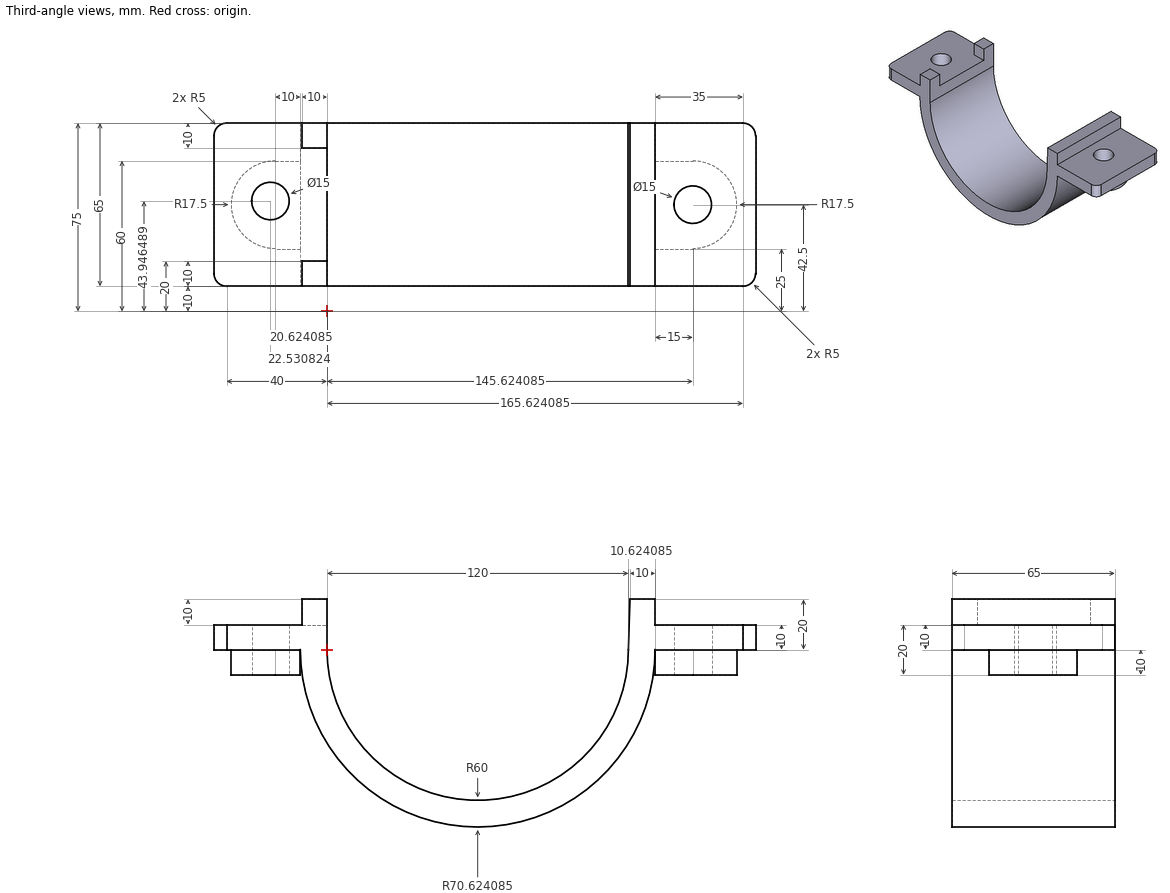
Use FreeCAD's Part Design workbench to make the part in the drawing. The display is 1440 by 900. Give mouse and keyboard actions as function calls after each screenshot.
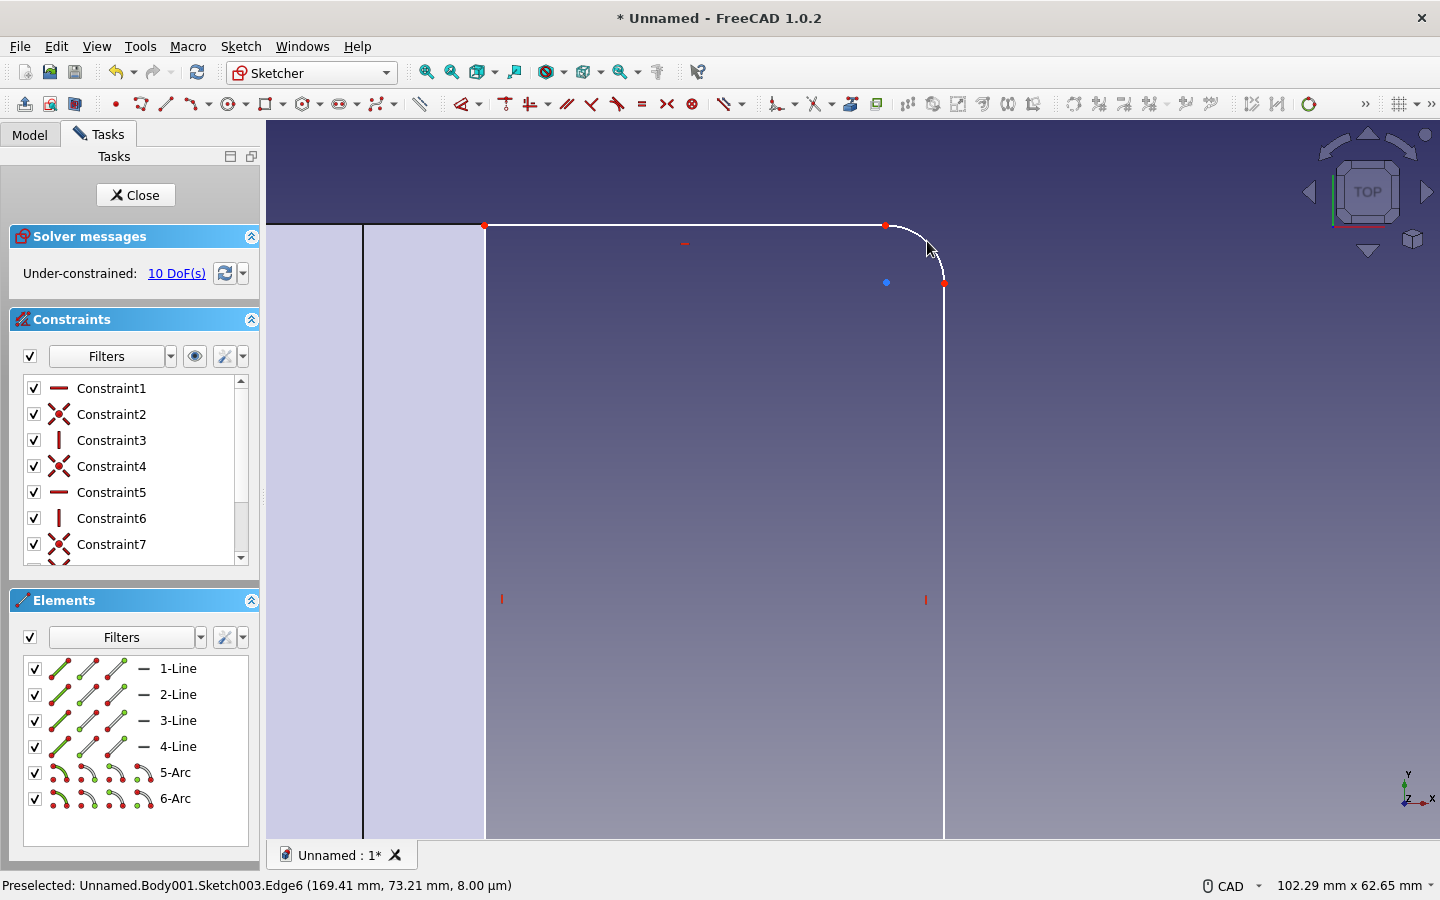
click(766, 225)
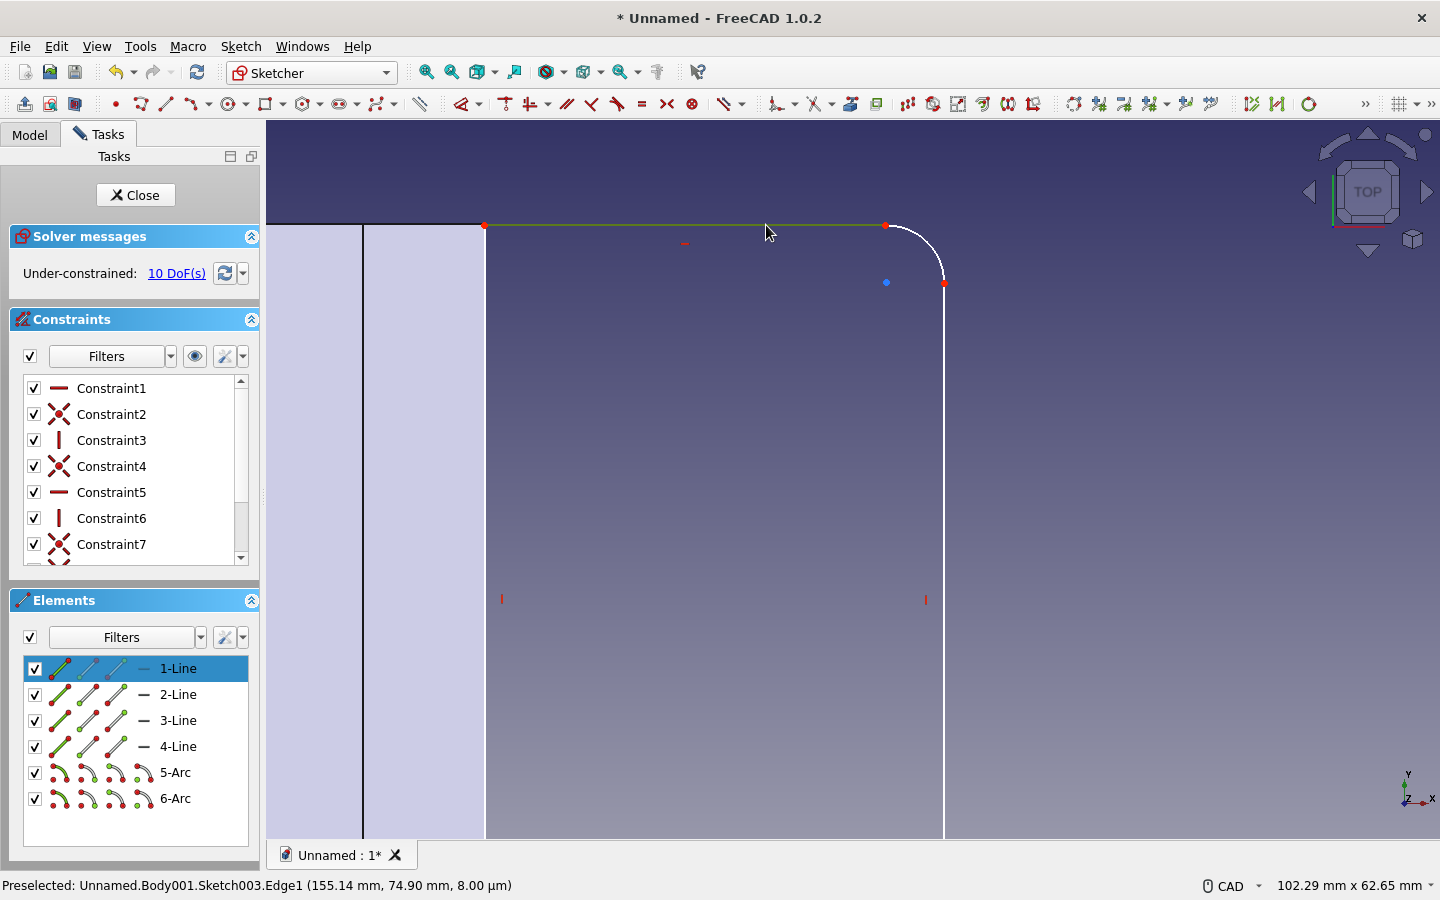
click(938, 257)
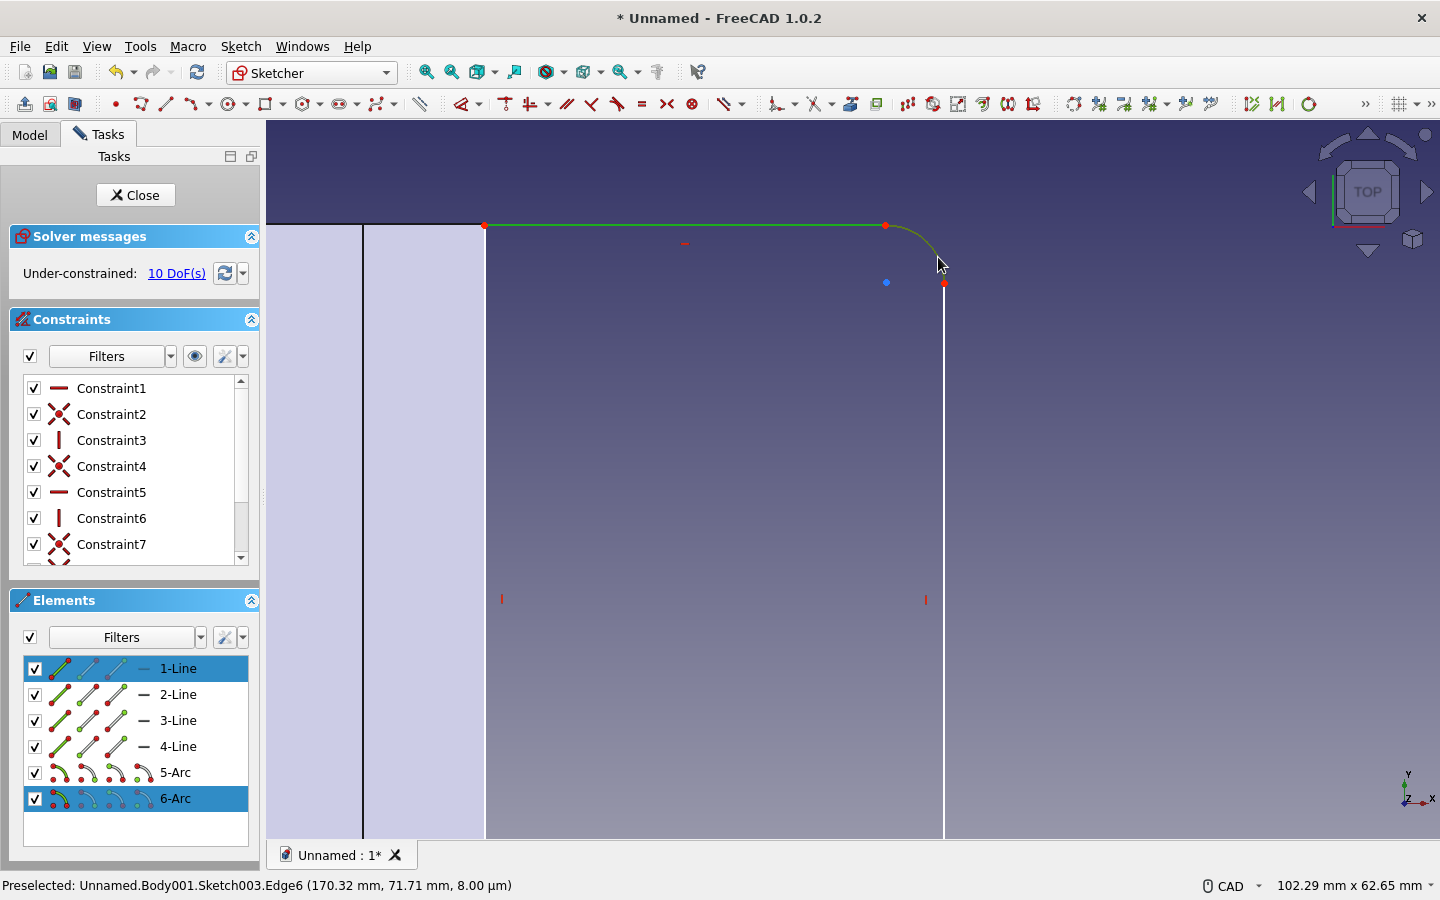
key(t)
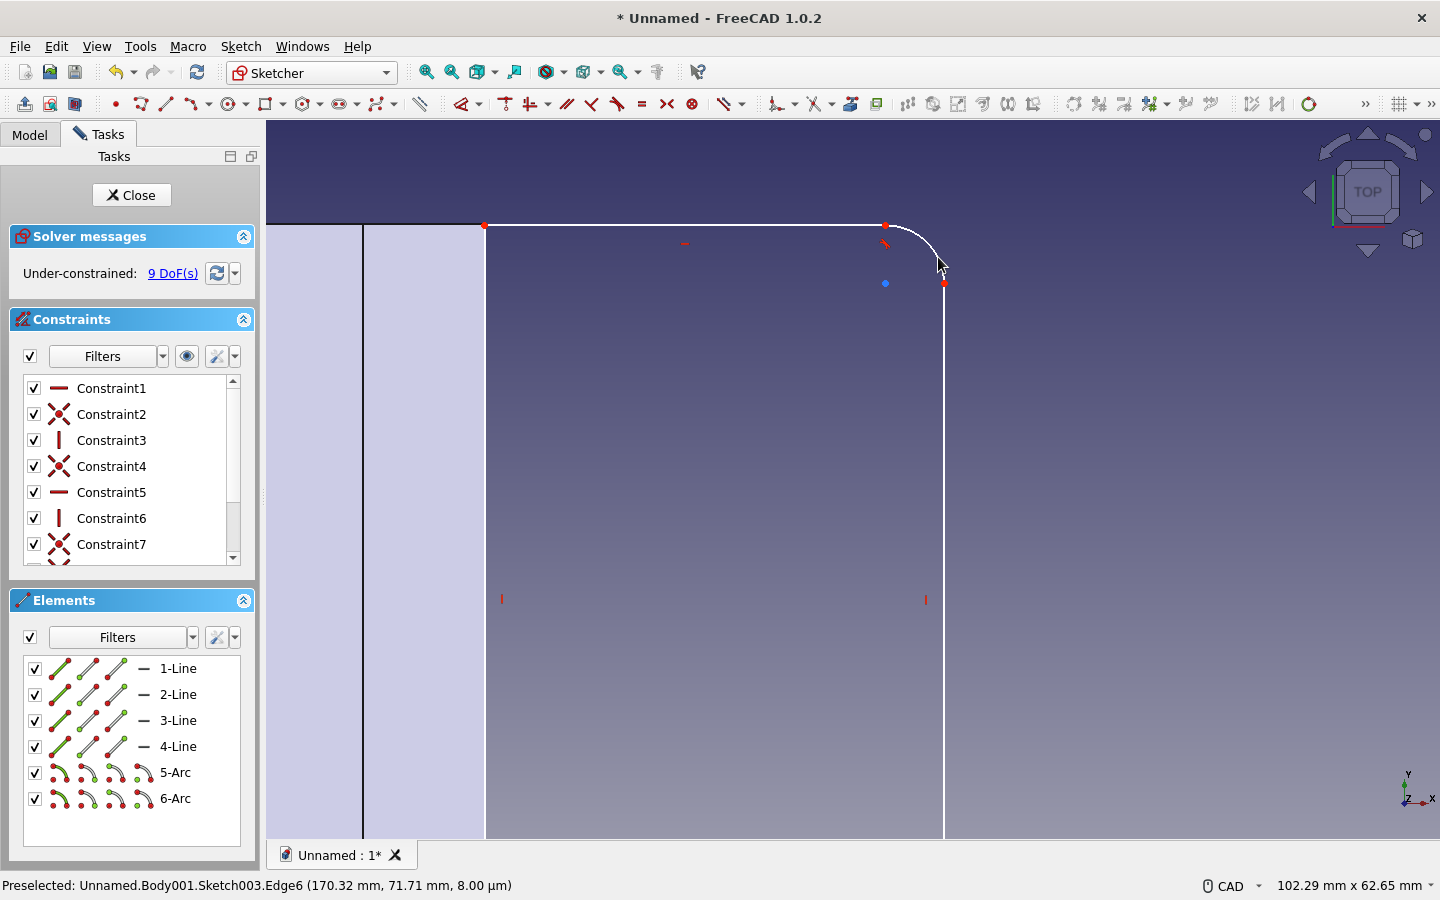
scroll(927, 240, down, 2)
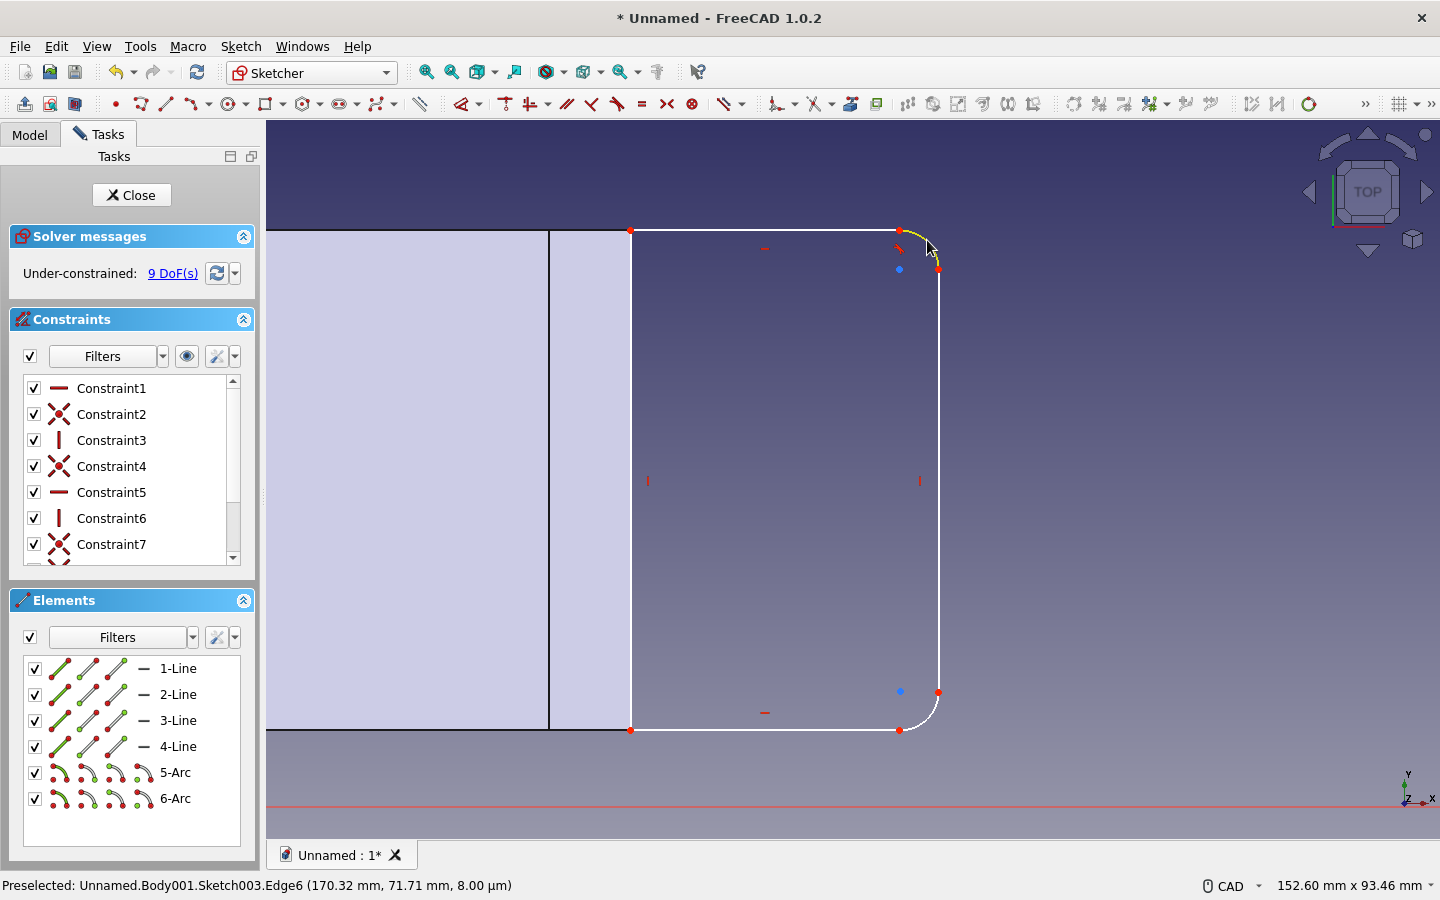
click(711, 730)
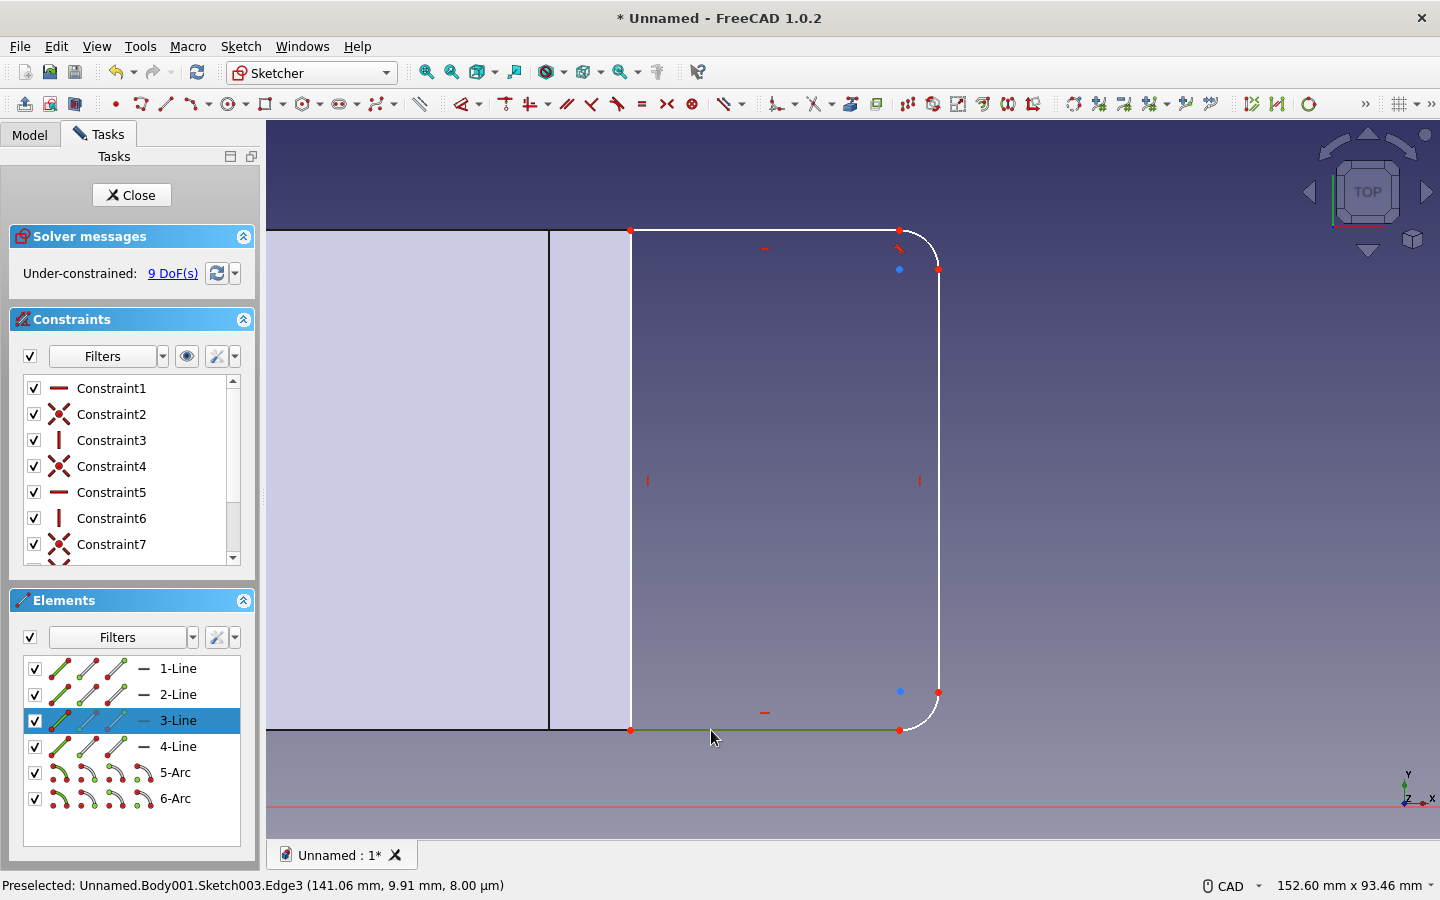
click(917, 726)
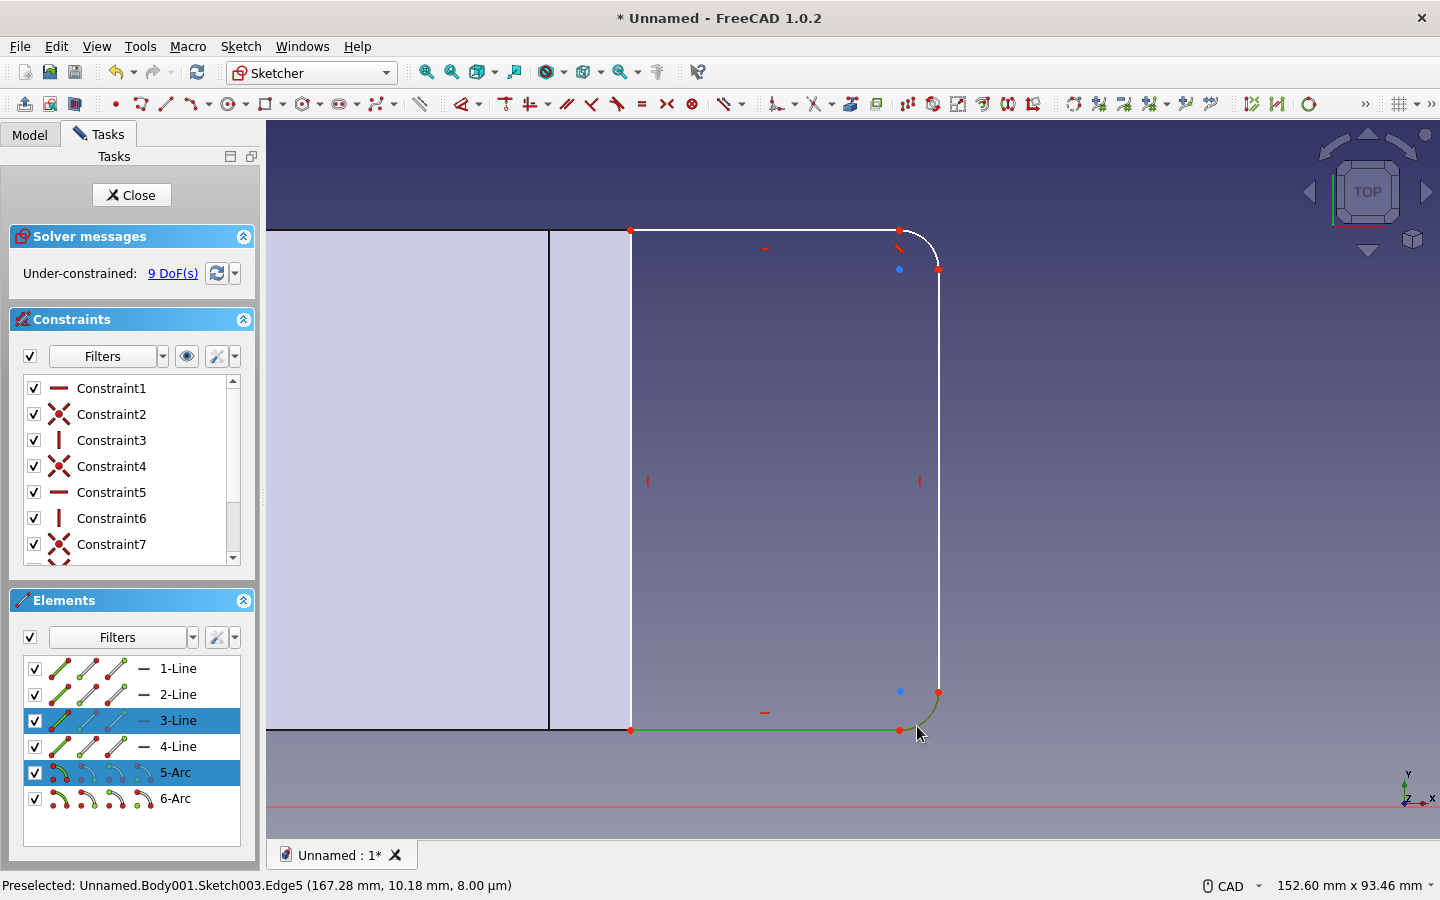
key(t)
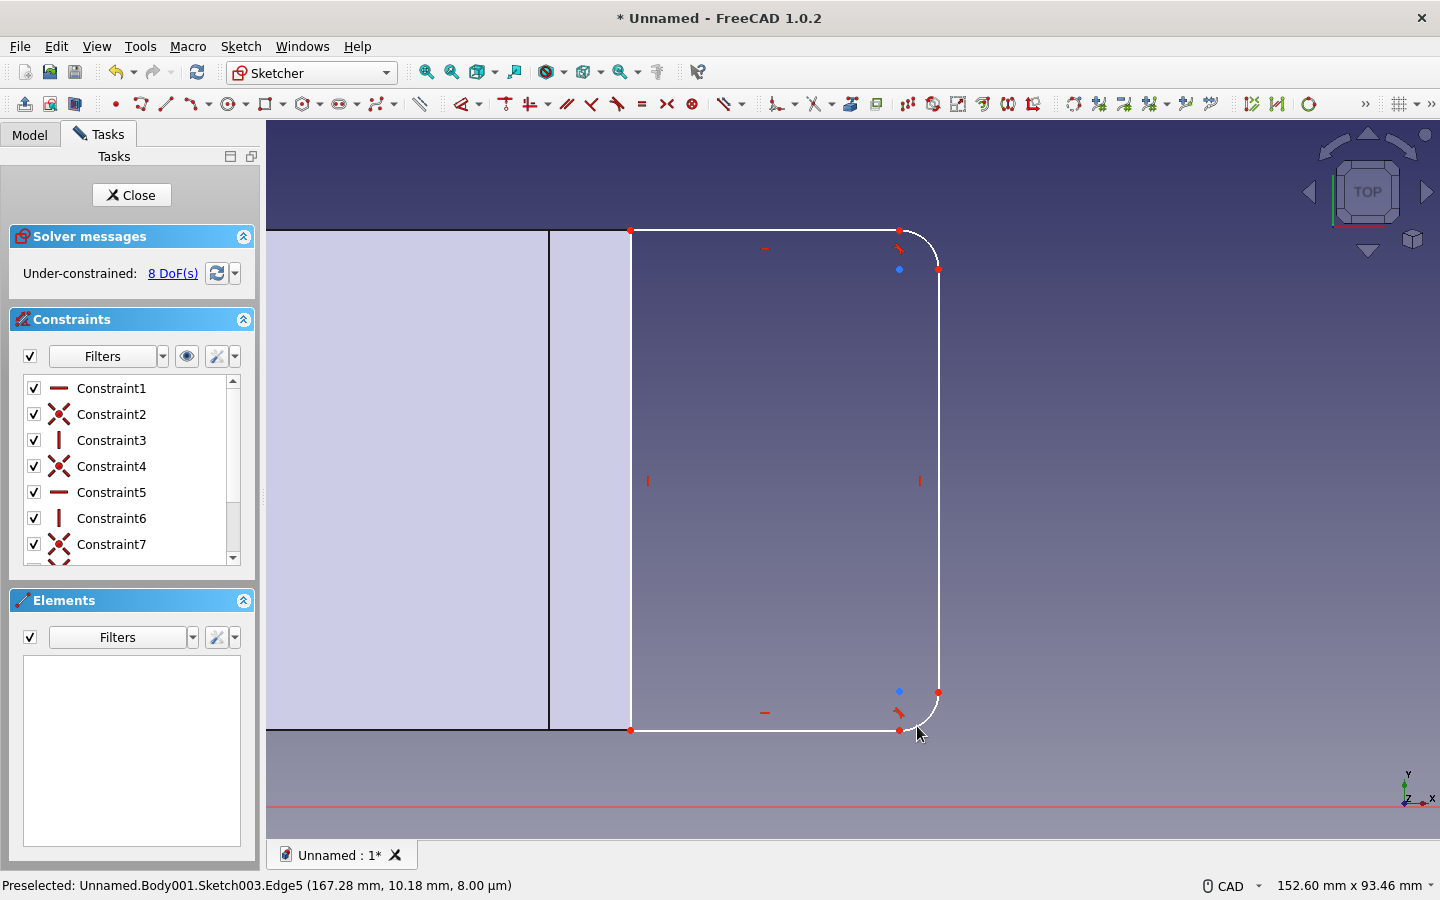
click(939, 565)